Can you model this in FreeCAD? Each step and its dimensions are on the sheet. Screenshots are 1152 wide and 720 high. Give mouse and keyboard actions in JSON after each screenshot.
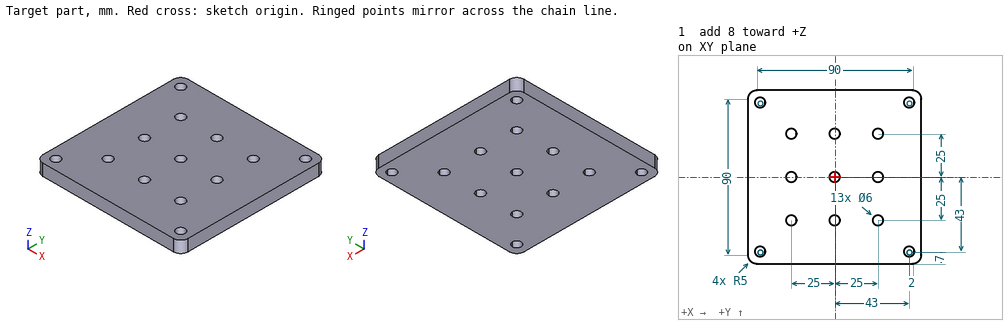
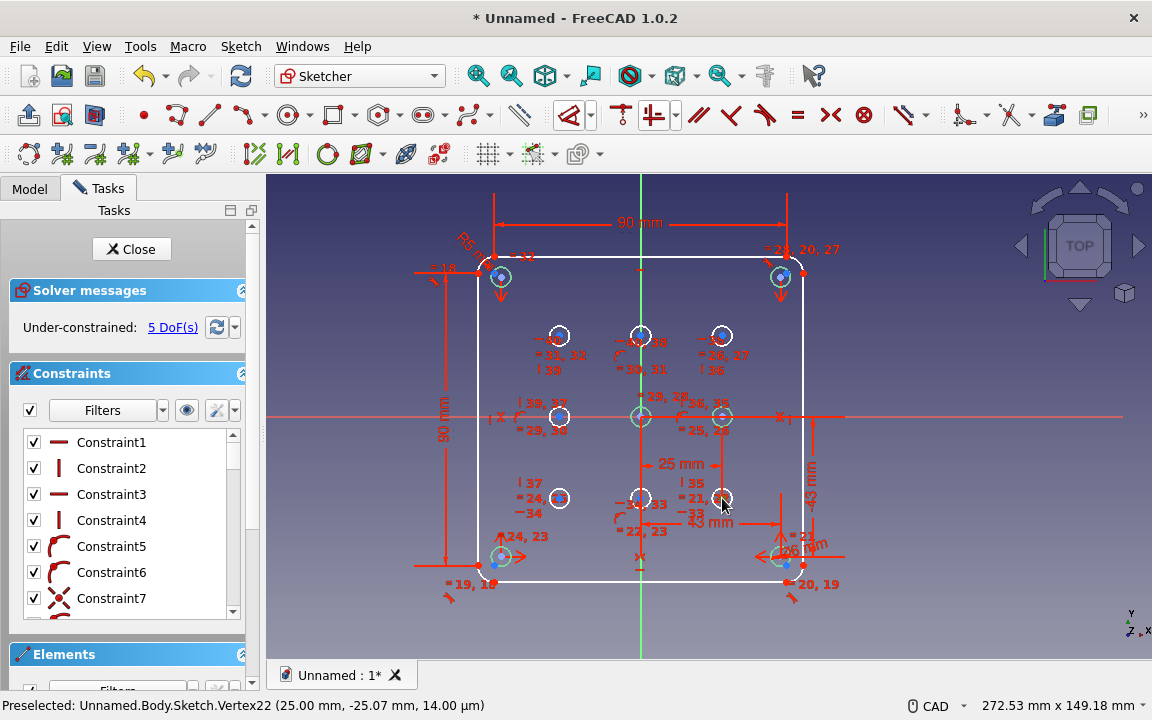
{"action": "left_click", "coordinate": [590, 116]}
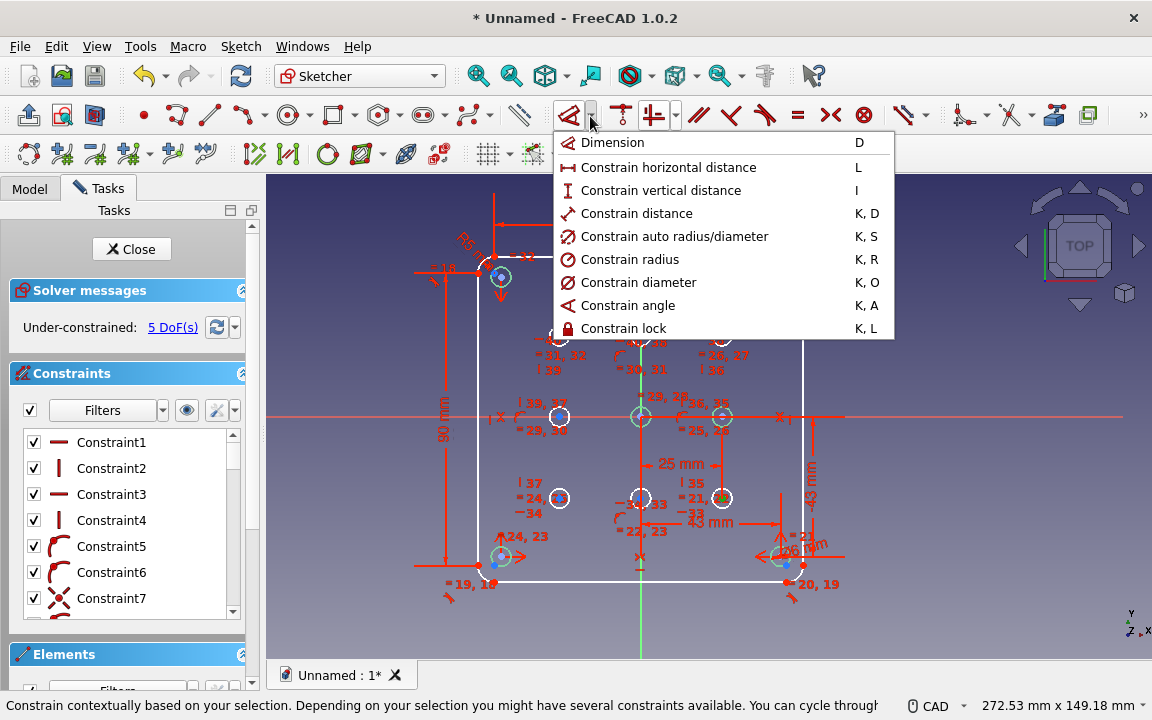
{"action": "left_click", "coordinate": [724, 190]}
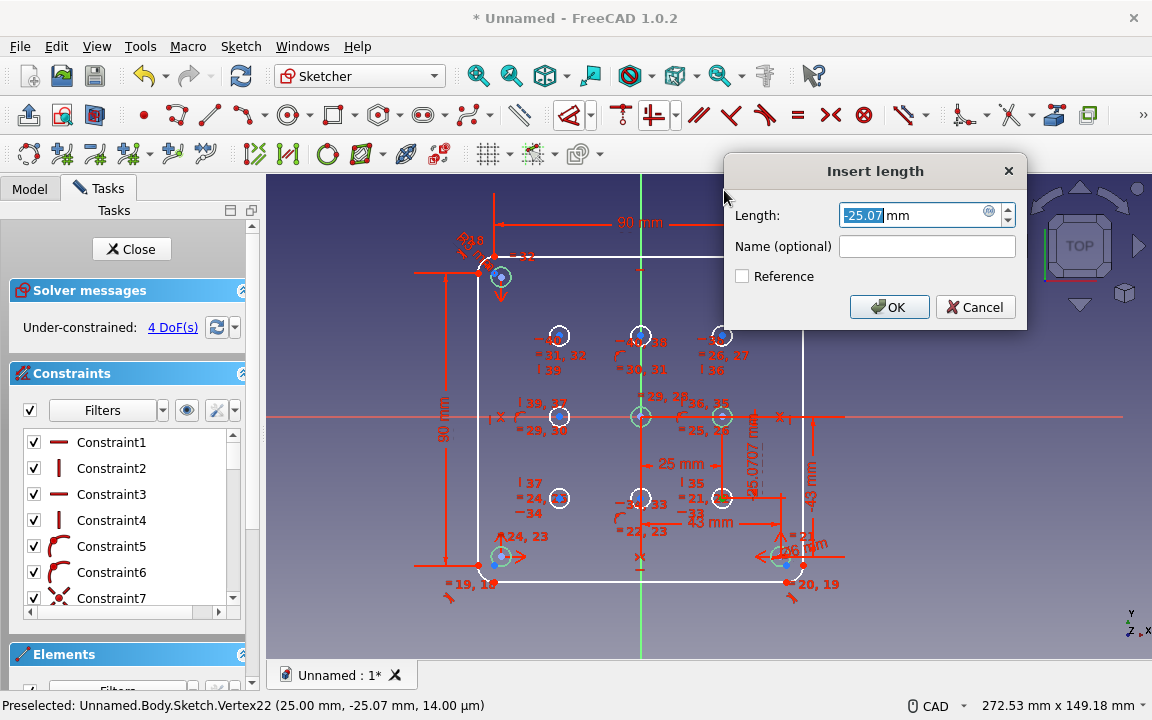
{"action": "type", "text": "-25"}
{"action": "key", "text": "Return"}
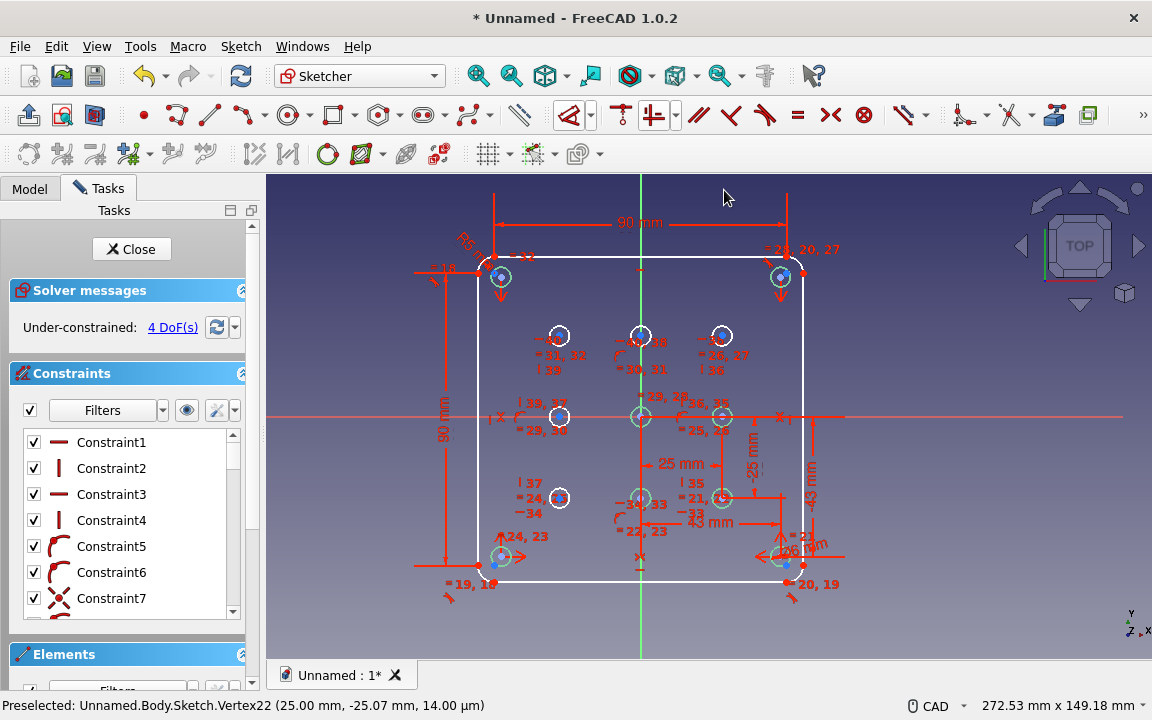
{"action": "left_click", "coordinate": [560, 498]}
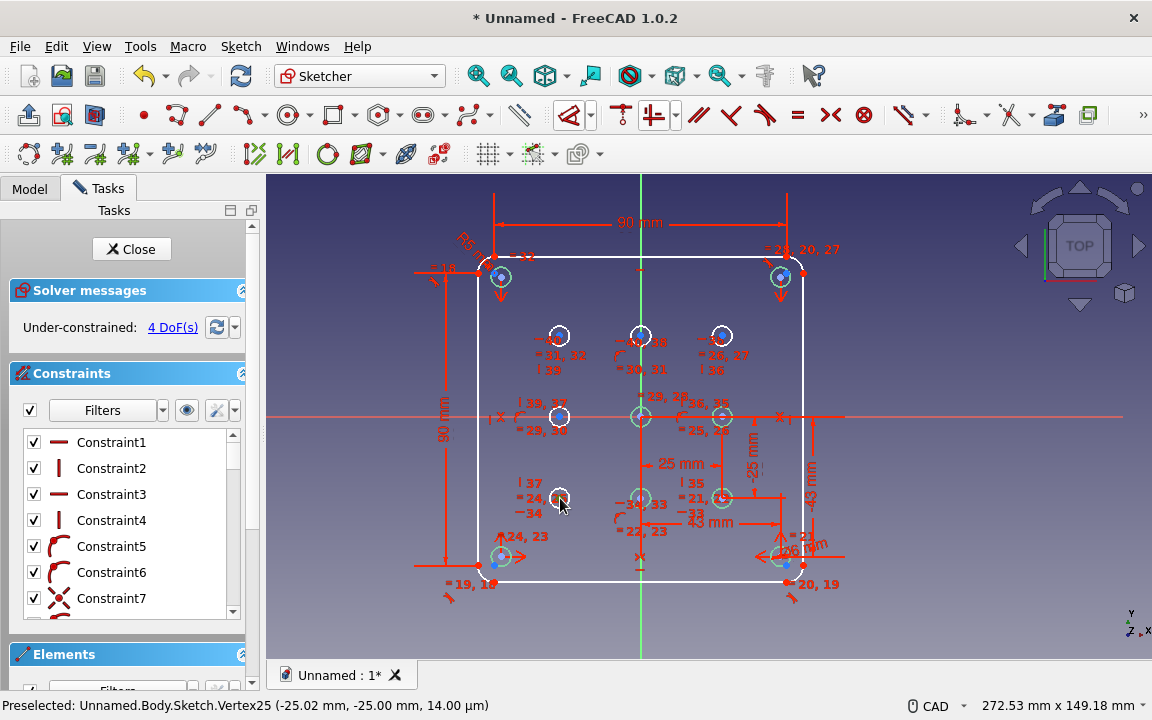
{"action": "key", "text": "l"}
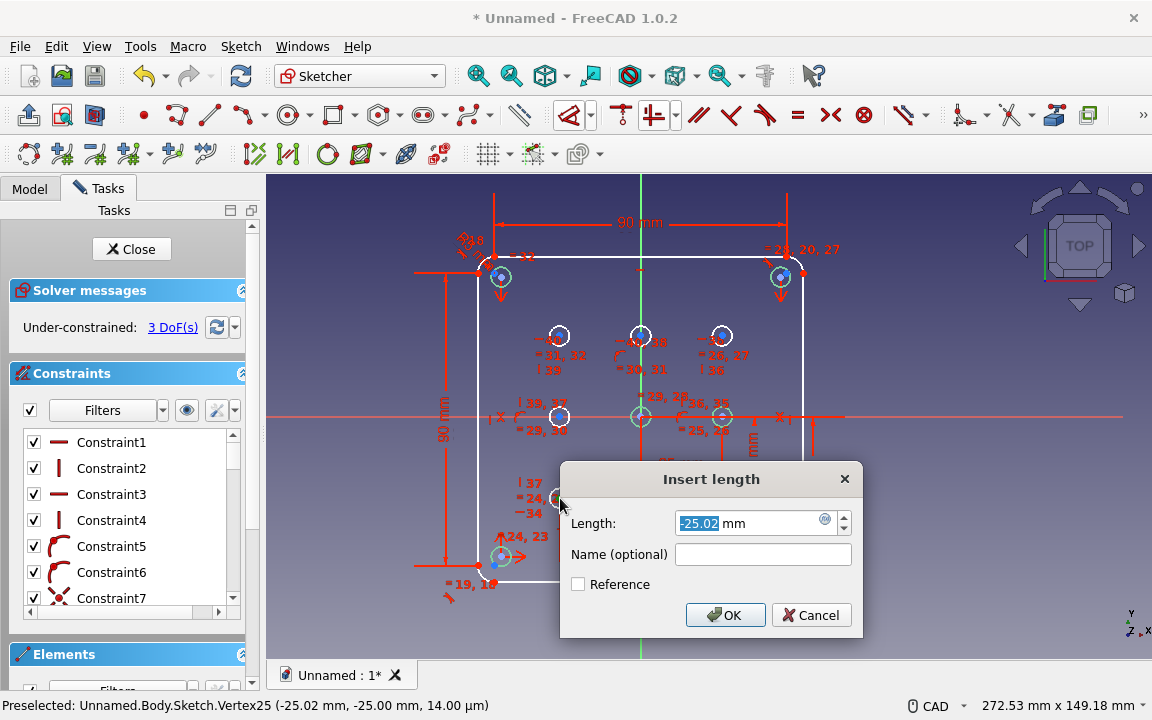
{"action": "type", "text": "-25"}
{"action": "key", "text": "Return"}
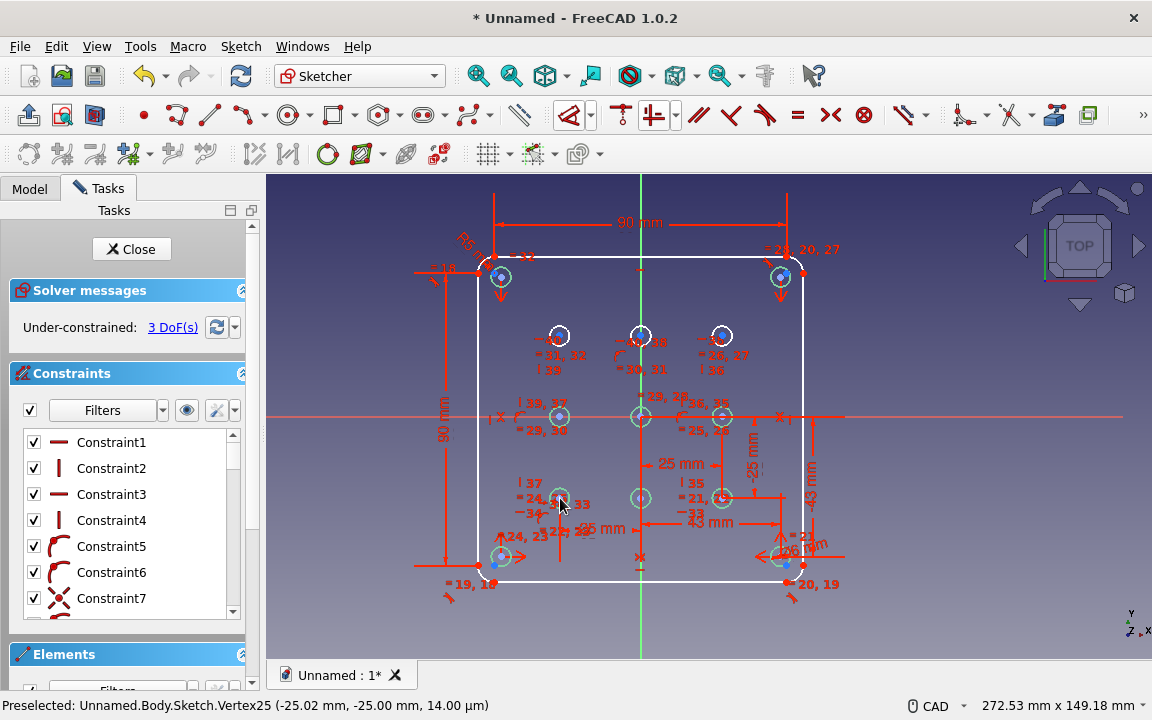
{"action": "left_click", "coordinate": [722, 336]}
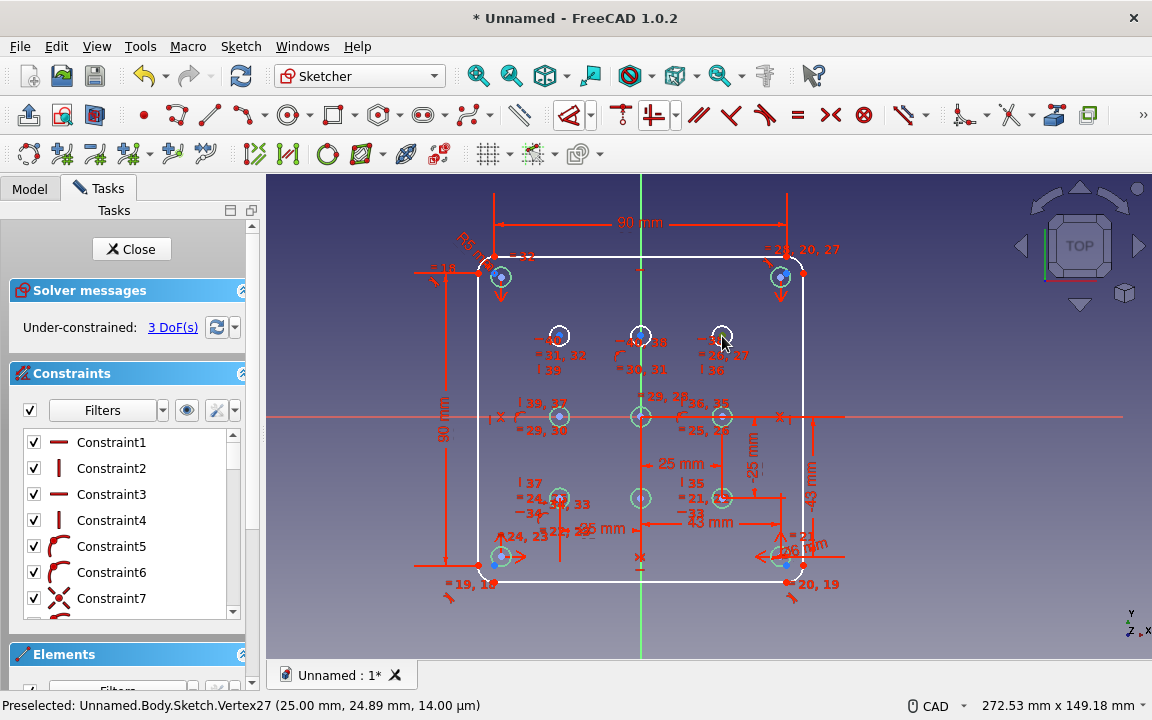
{"action": "key", "text": "i"}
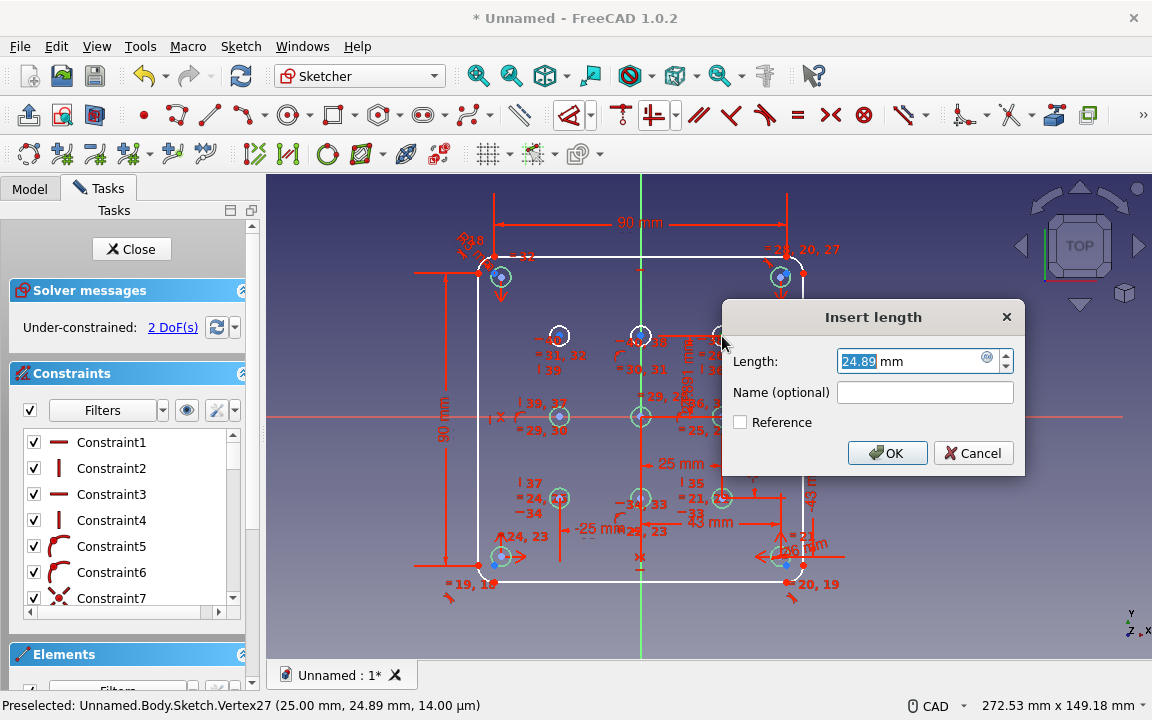
{"action": "type", "text": "25"}
{"action": "key", "text": "Return"}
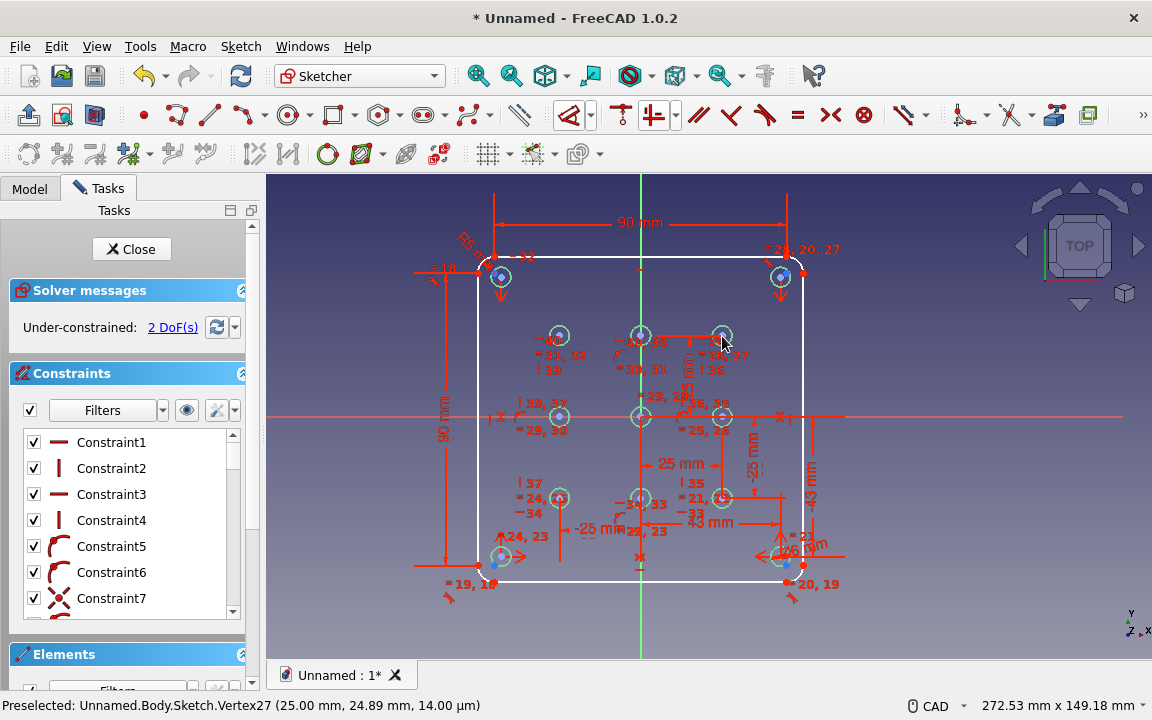
{"action": "scroll", "coordinate": [787, 582], "scroll_direction": "up", "scroll_amount": 10}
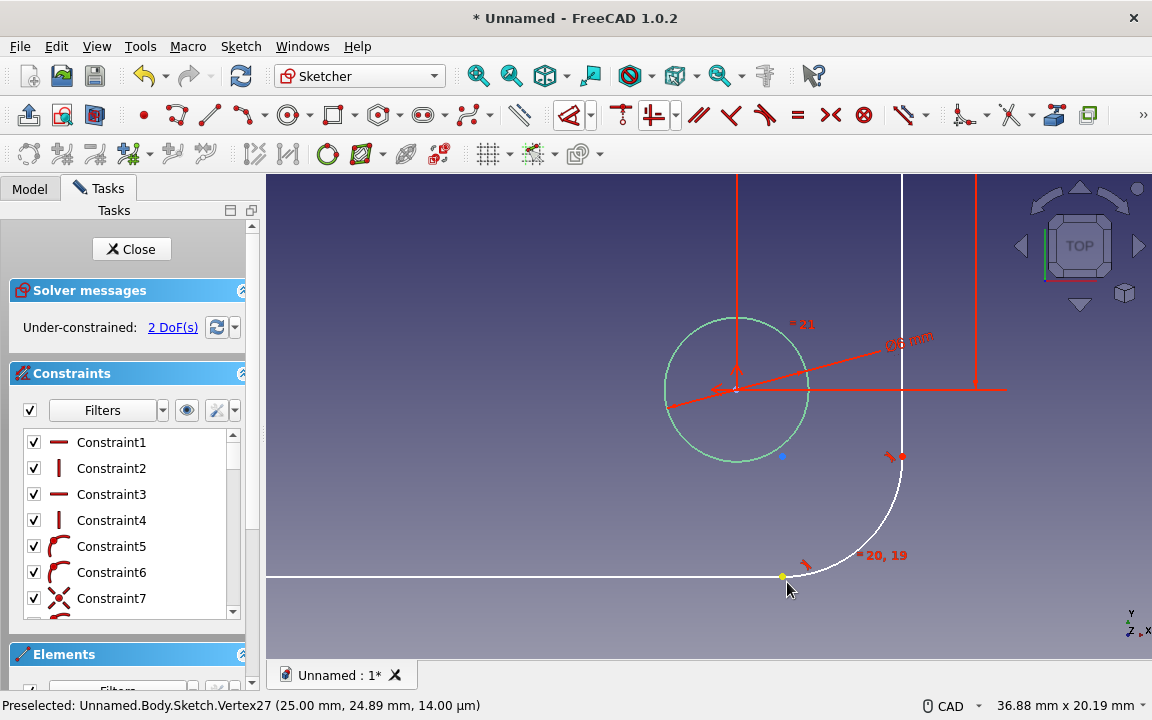
{"action": "left_click", "coordinate": [782, 577]}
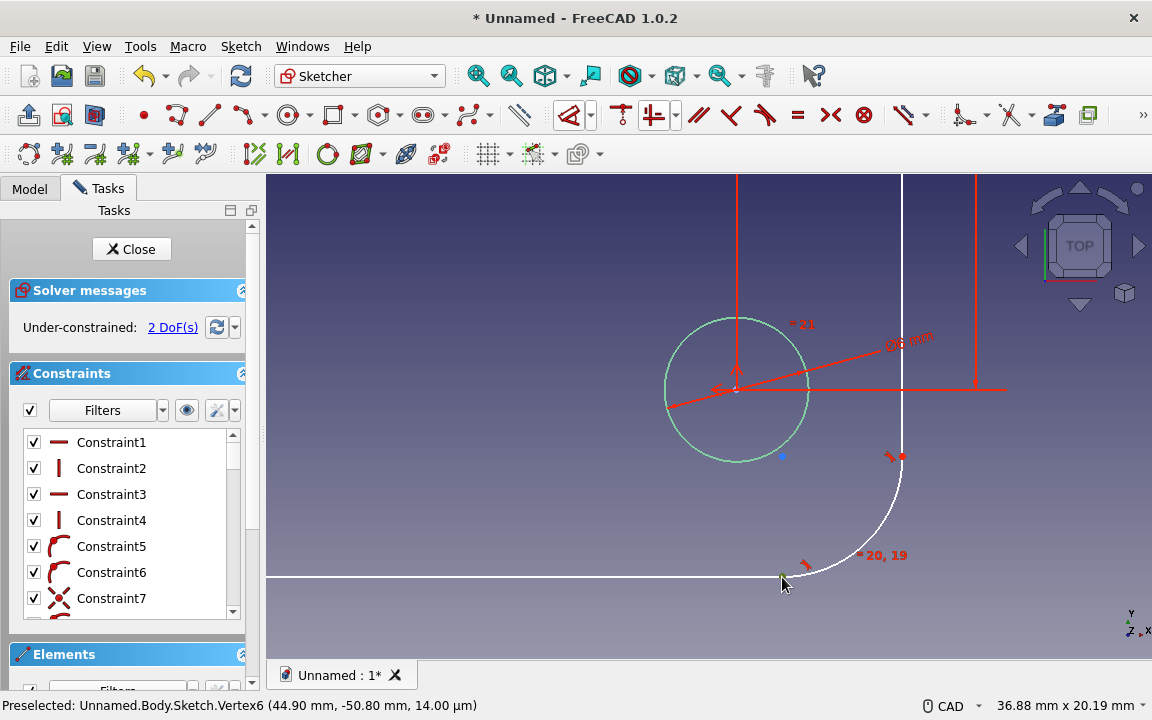
{"action": "left_click", "coordinate": [737, 390]}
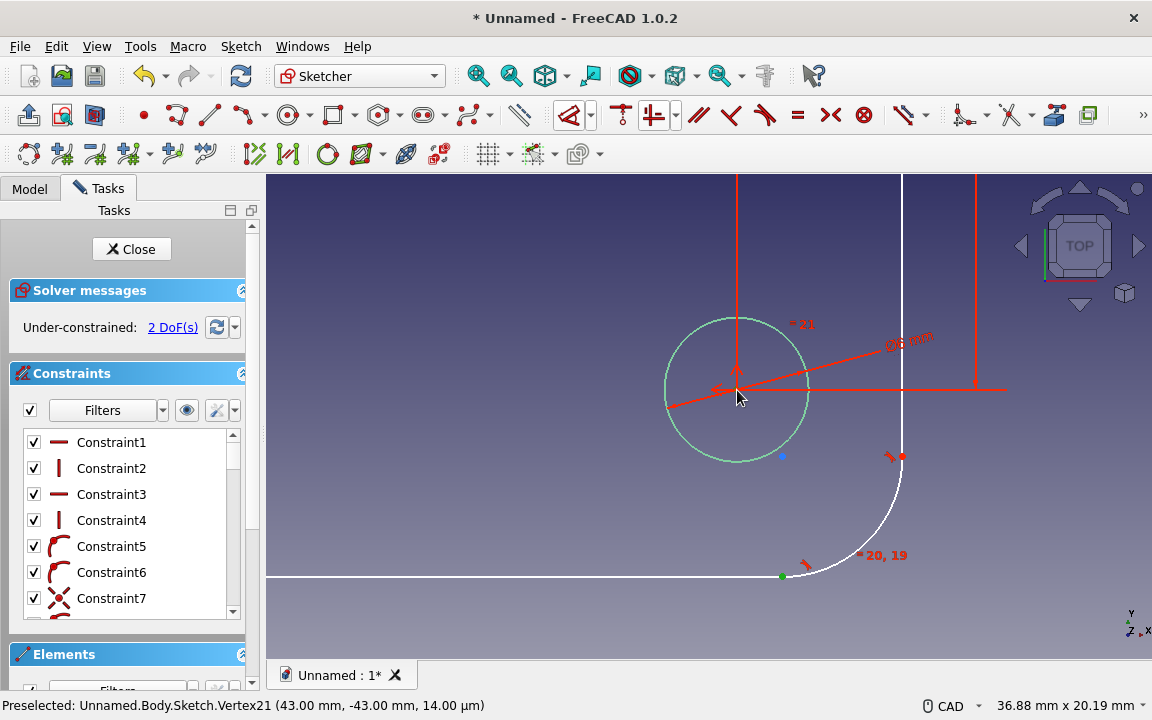
{"action": "key", "text": "l"}